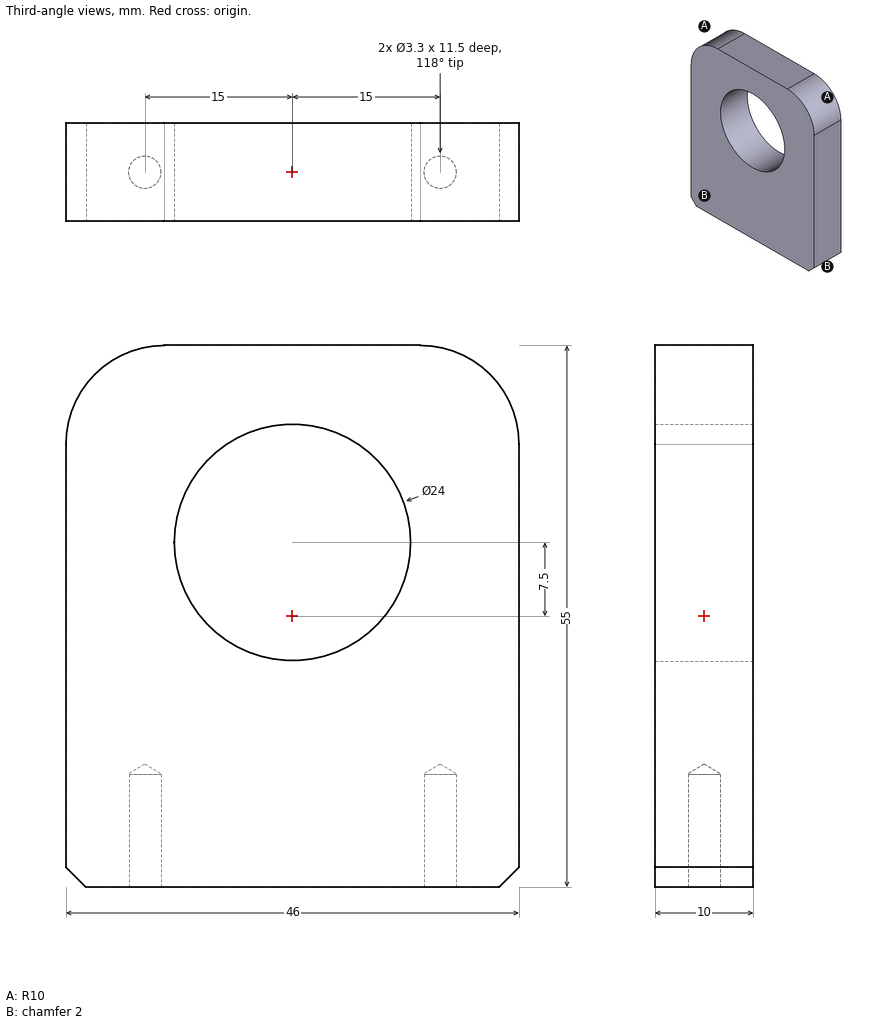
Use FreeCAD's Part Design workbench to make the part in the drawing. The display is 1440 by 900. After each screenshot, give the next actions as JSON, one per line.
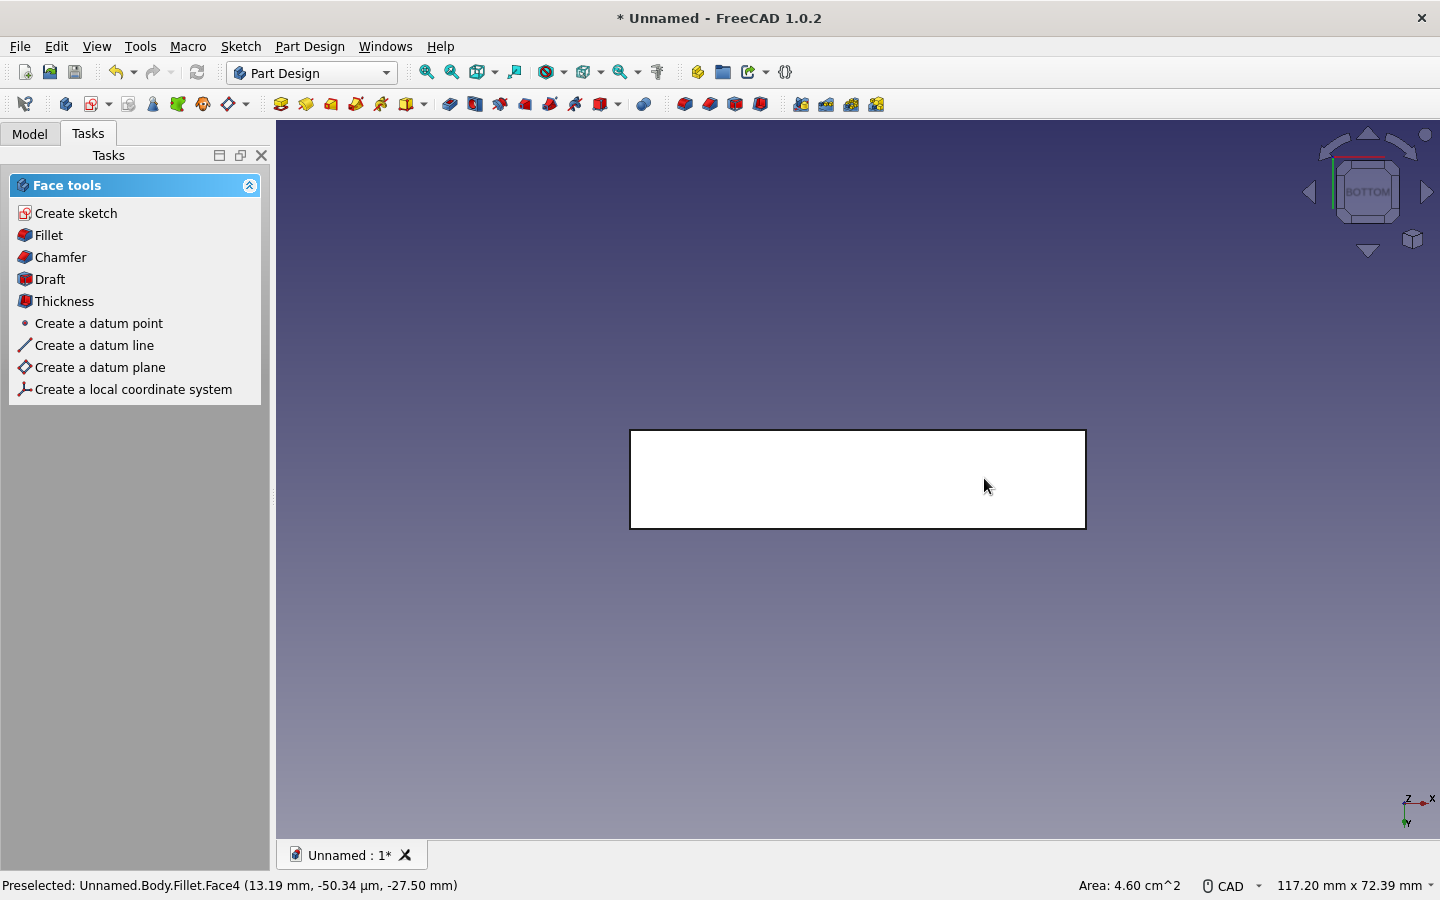
{"action": "left_click", "coordinate": [90, 104]}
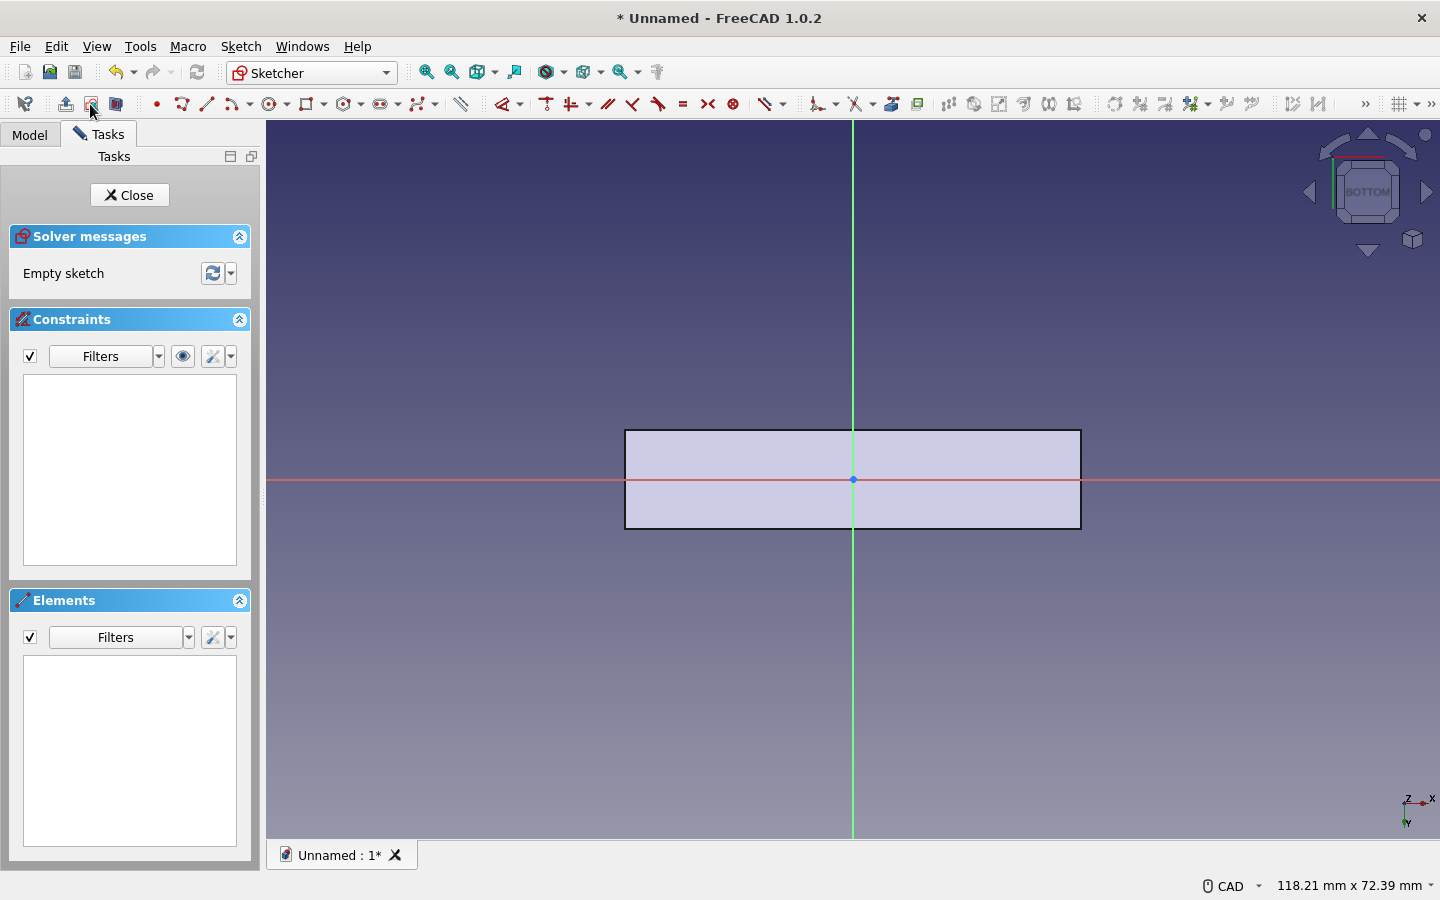
{"action": "scroll", "coordinate": [909, 479], "scroll_direction": "up", "scroll_amount": 4}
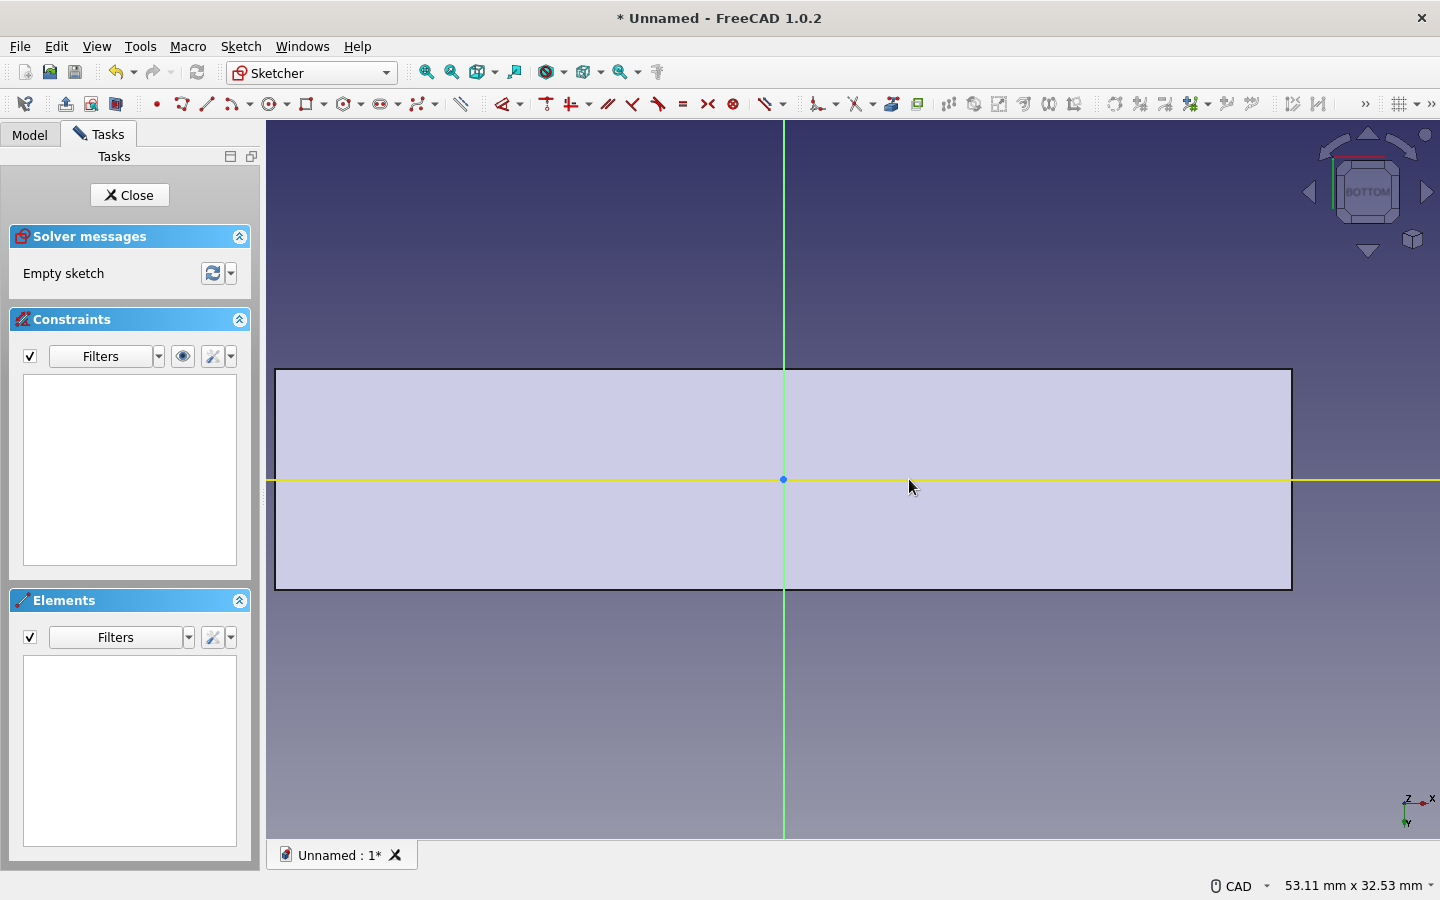
{"action": "left_click", "coordinate": [268, 104]}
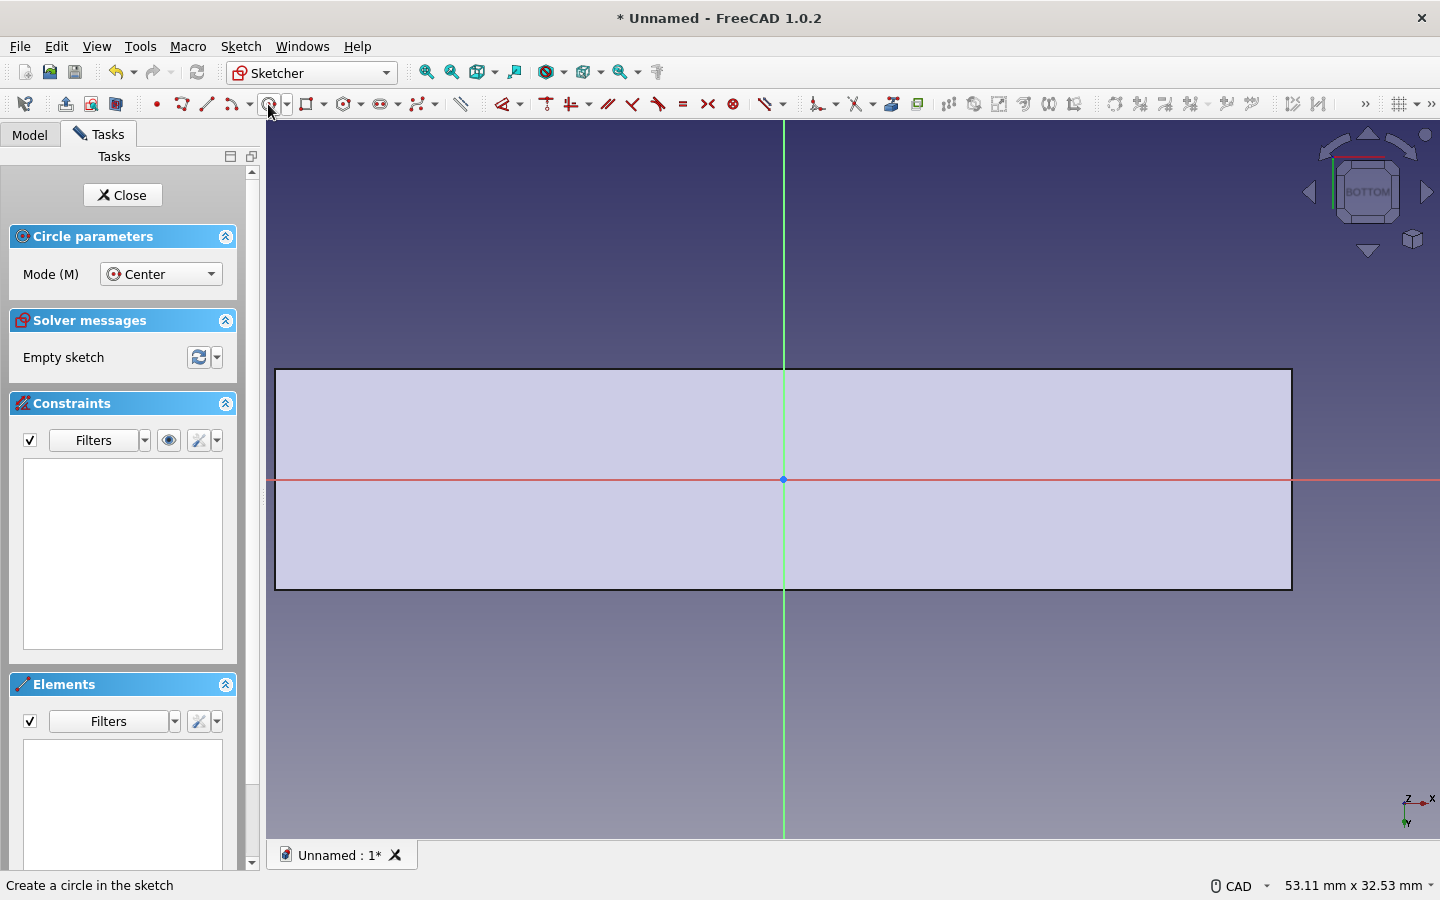
{"action": "left_click", "coordinate": [1115, 479]}
{"action": "left_click", "coordinate": [1141, 454]}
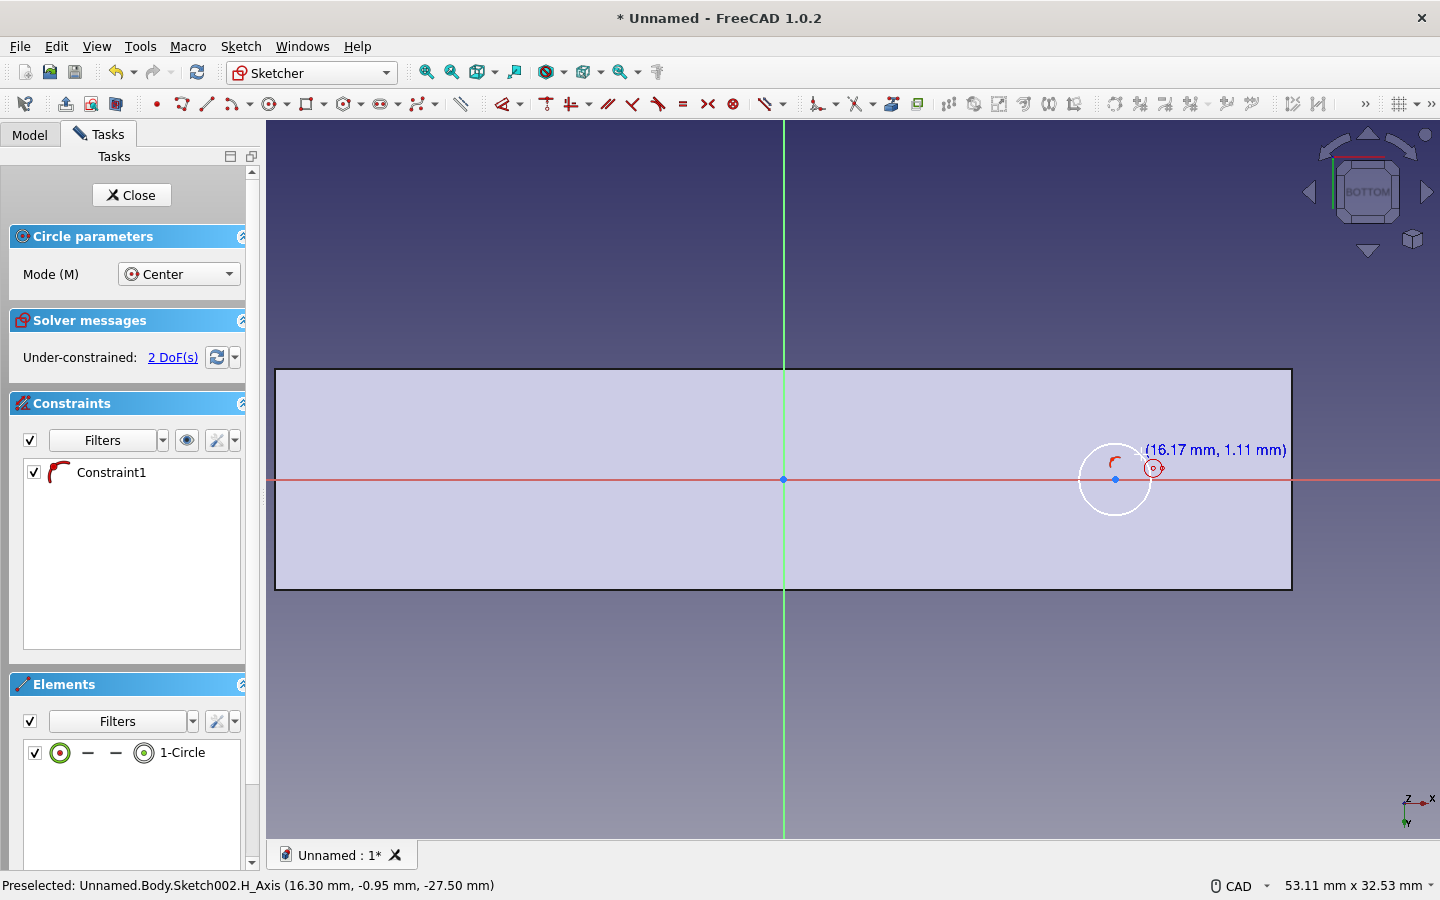
{"action": "left_click", "coordinate": [452, 479]}
{"action": "left_click", "coordinate": [478, 454]}
{"action": "key", "text": "Escape"}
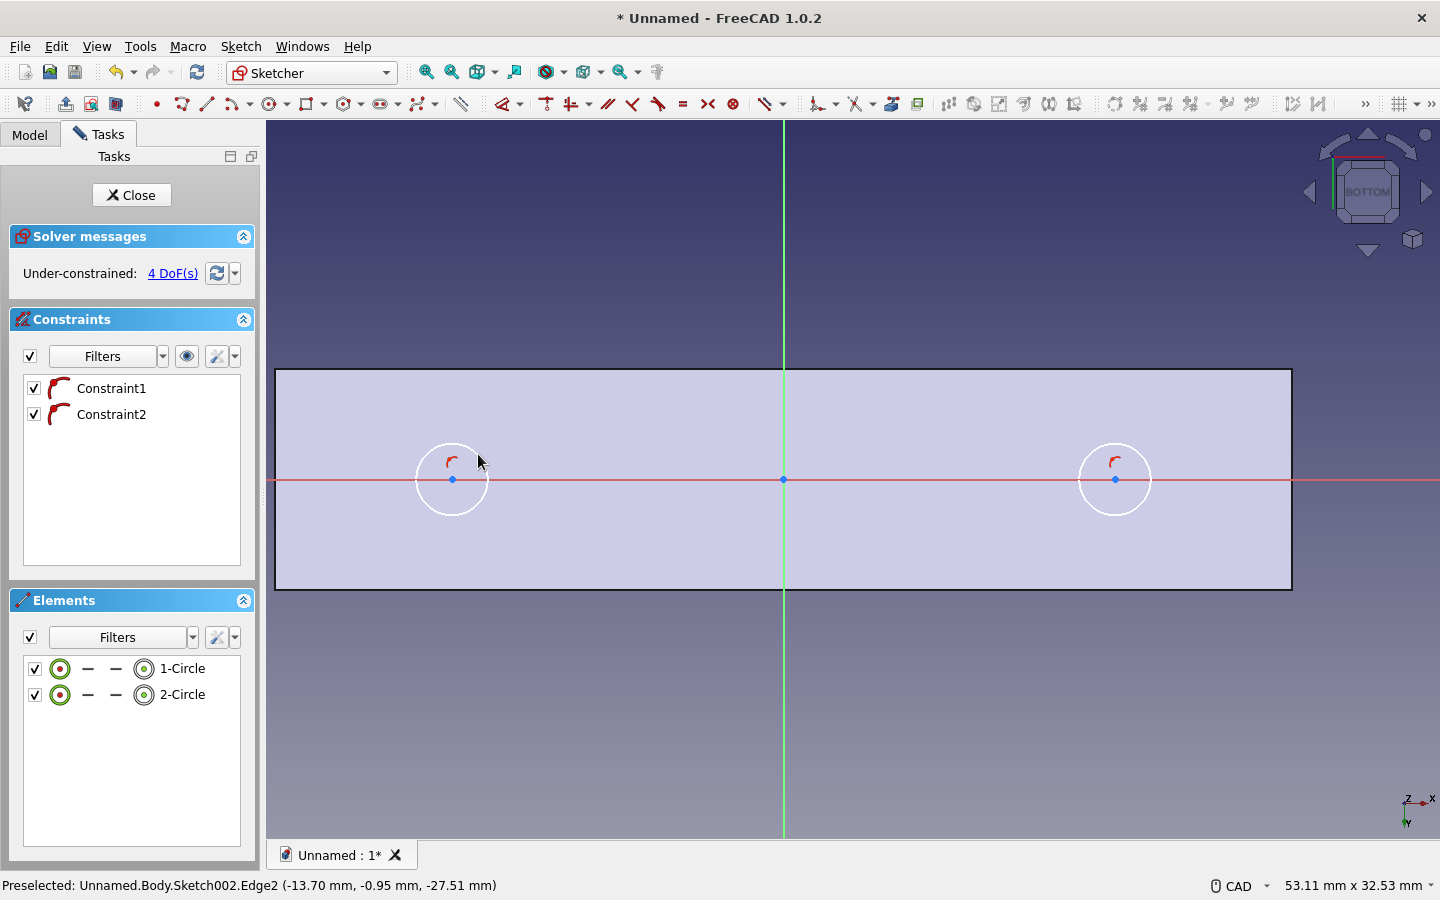
{"action": "left_click", "coordinate": [1140, 454]}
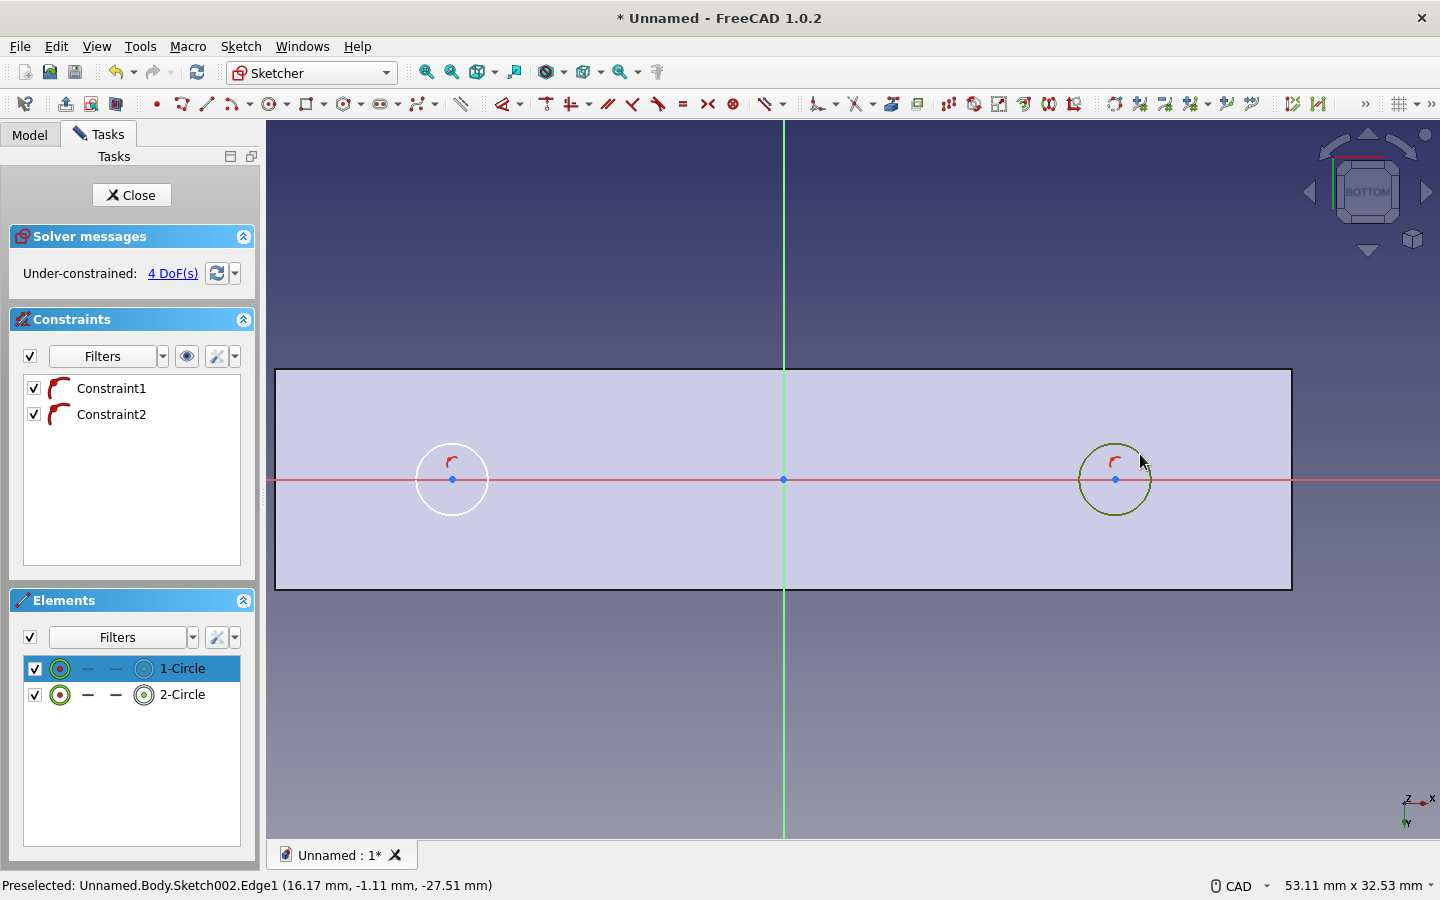
{"action": "left_click", "coordinate": [477, 454]}